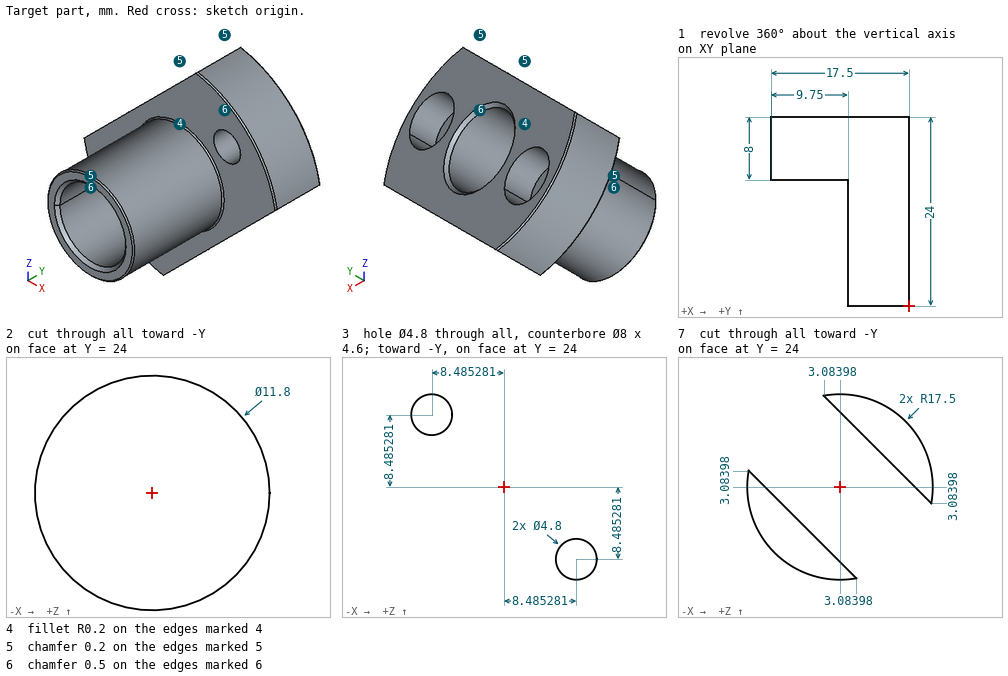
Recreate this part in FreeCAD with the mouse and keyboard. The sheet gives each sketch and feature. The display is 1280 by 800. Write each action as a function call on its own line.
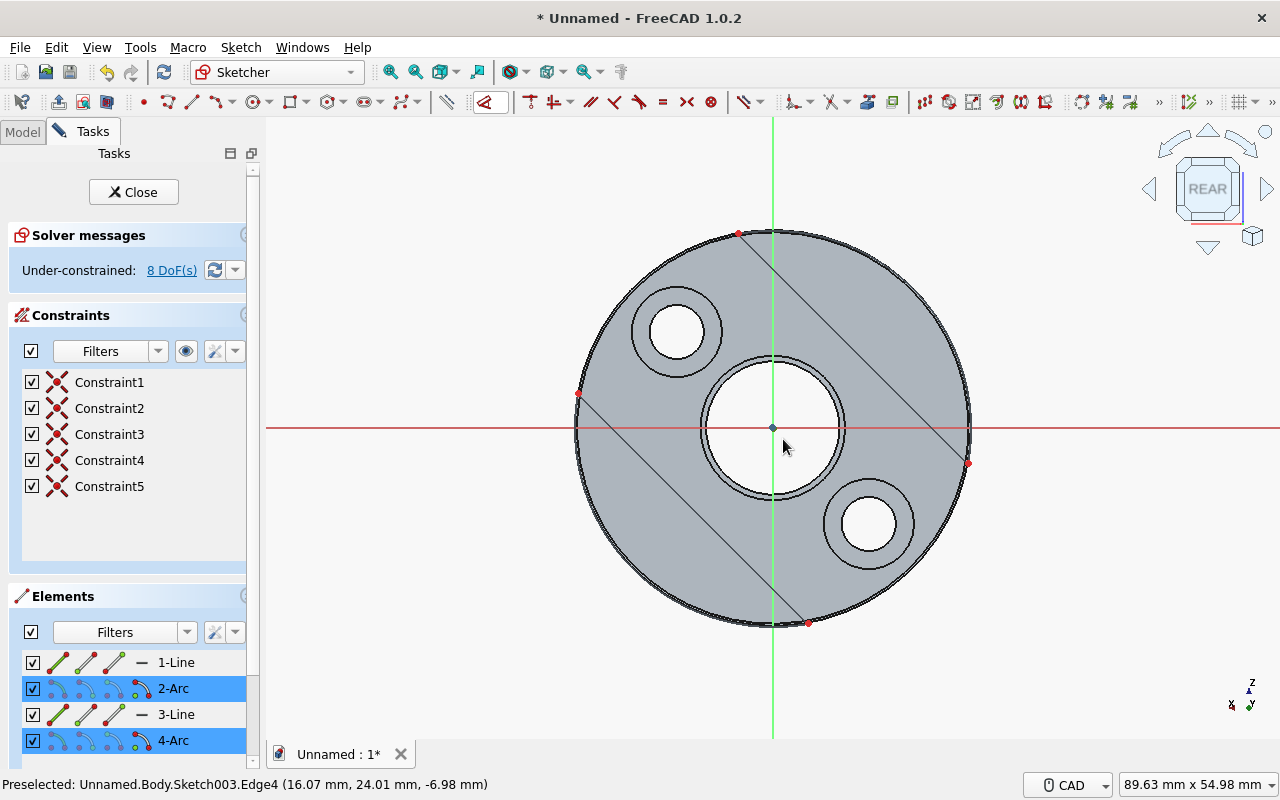
key(c)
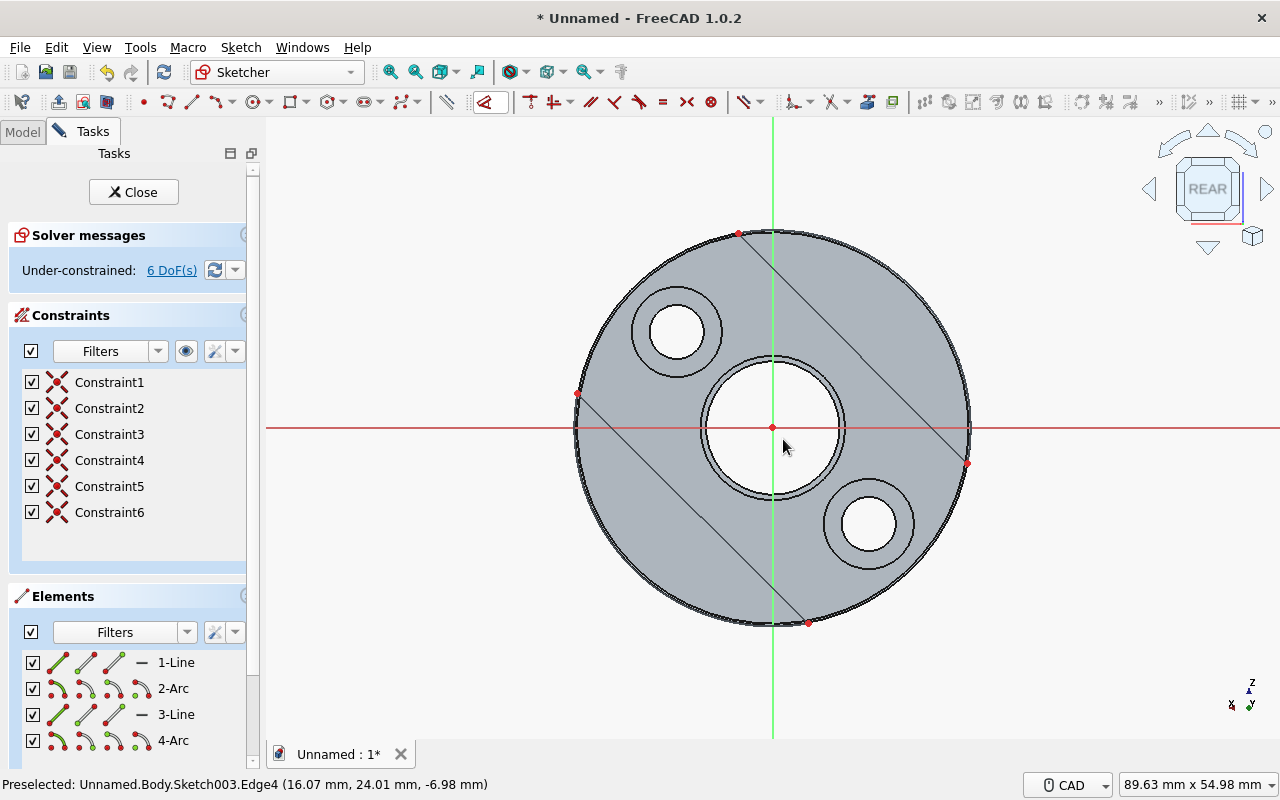
click(955, 352)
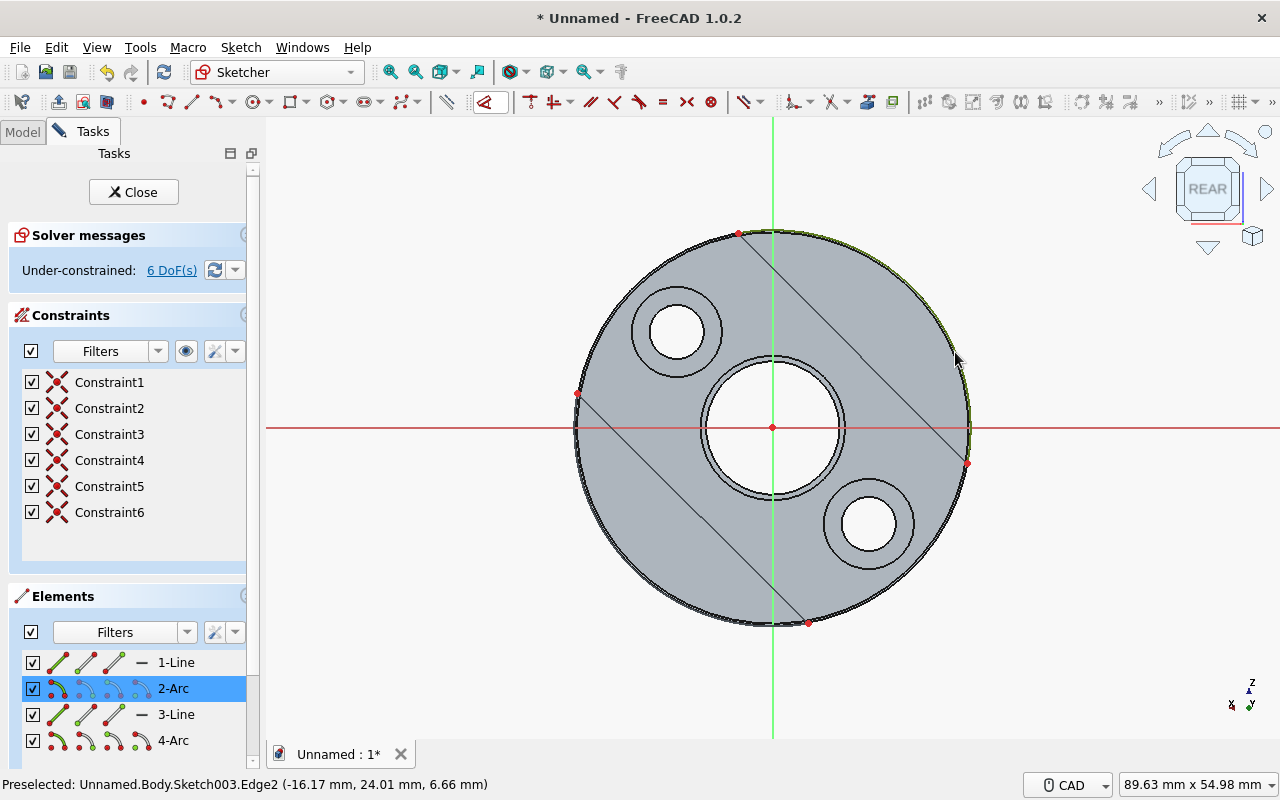
click(590, 506)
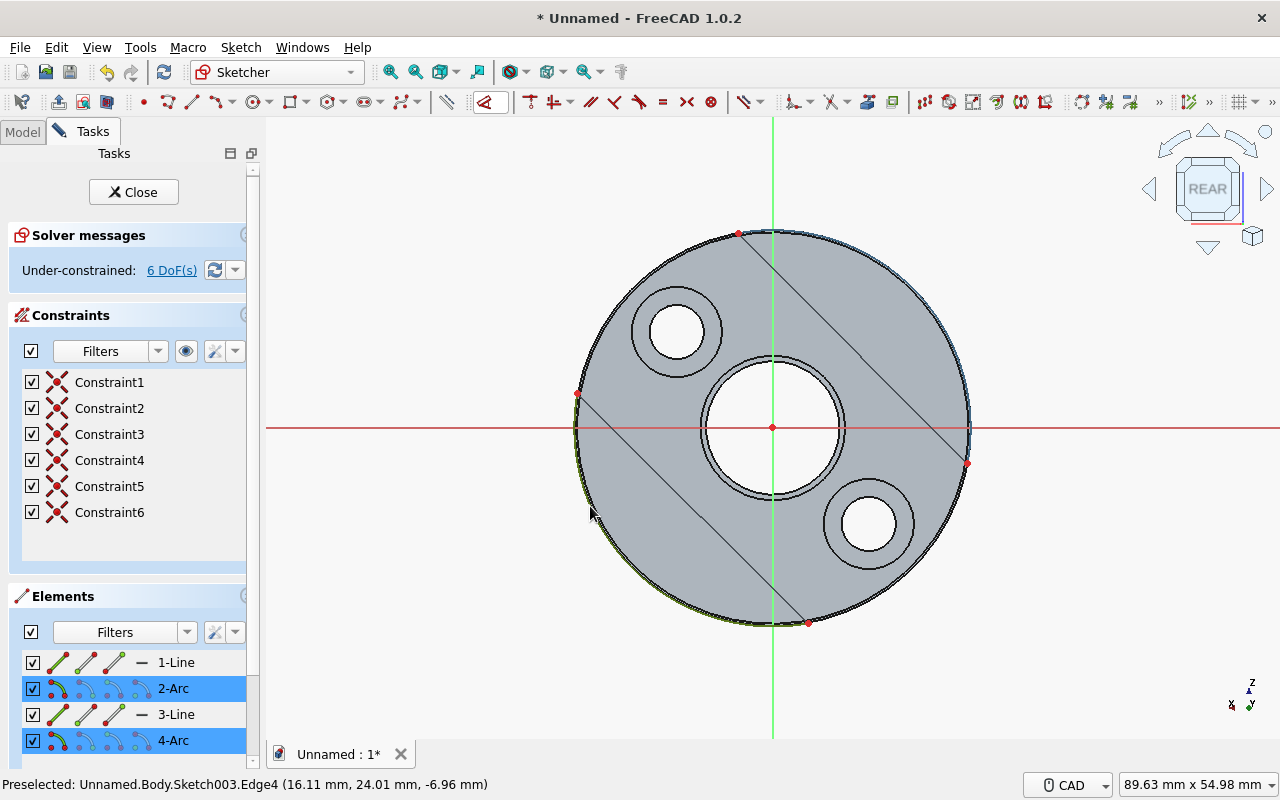
key(e)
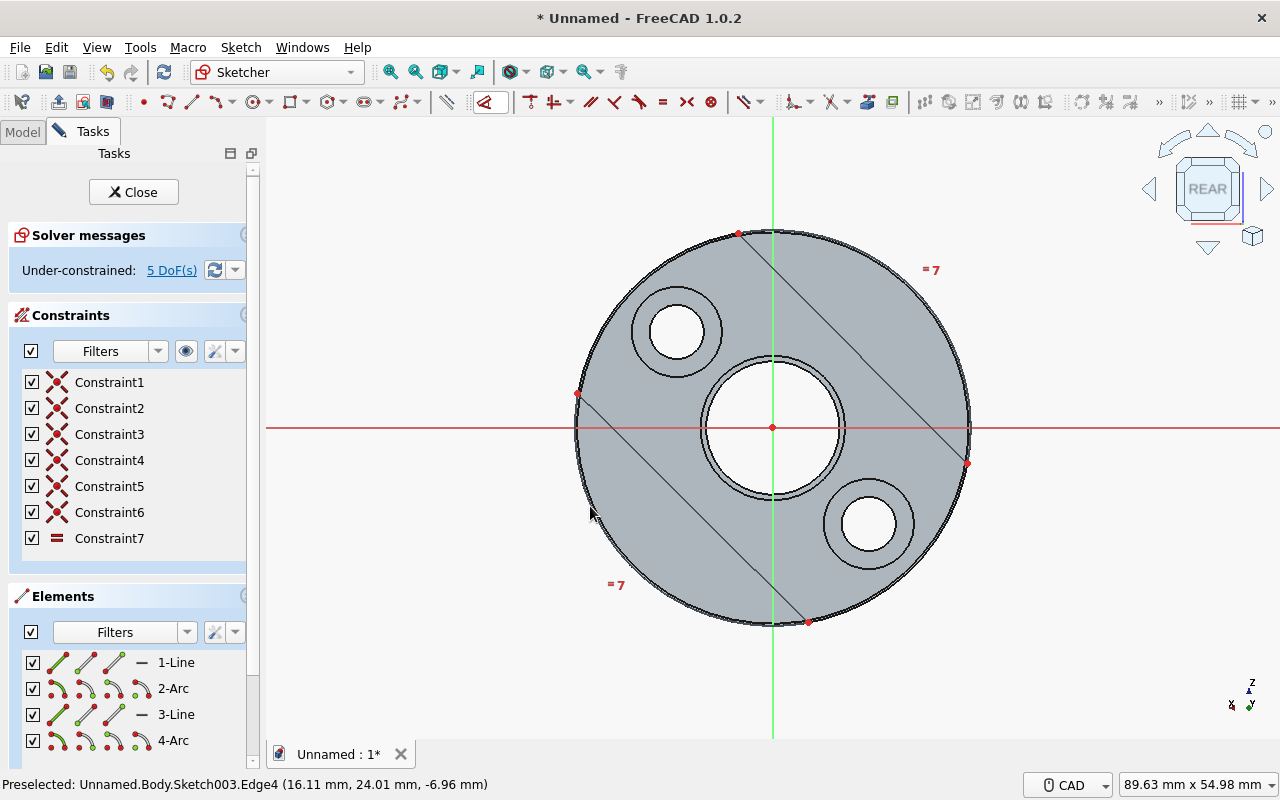
click(955, 352)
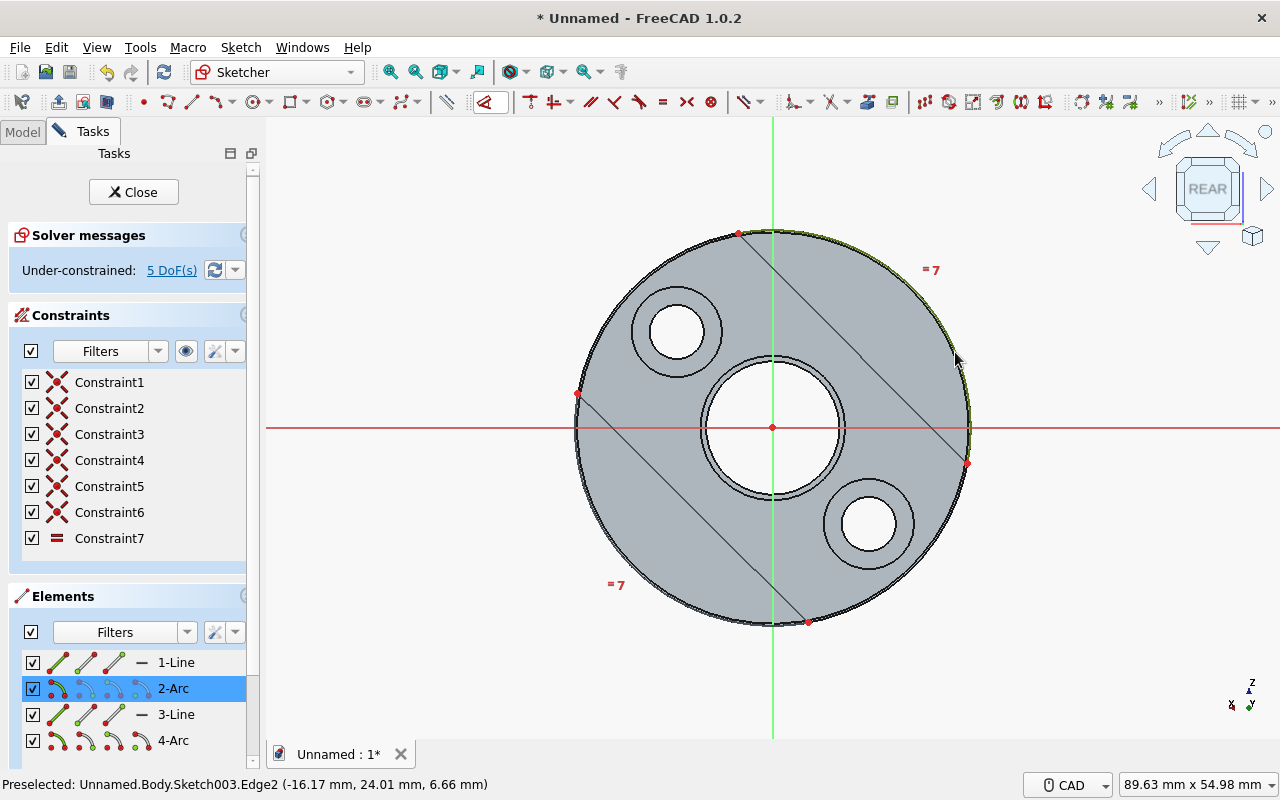
key(k)
key(r)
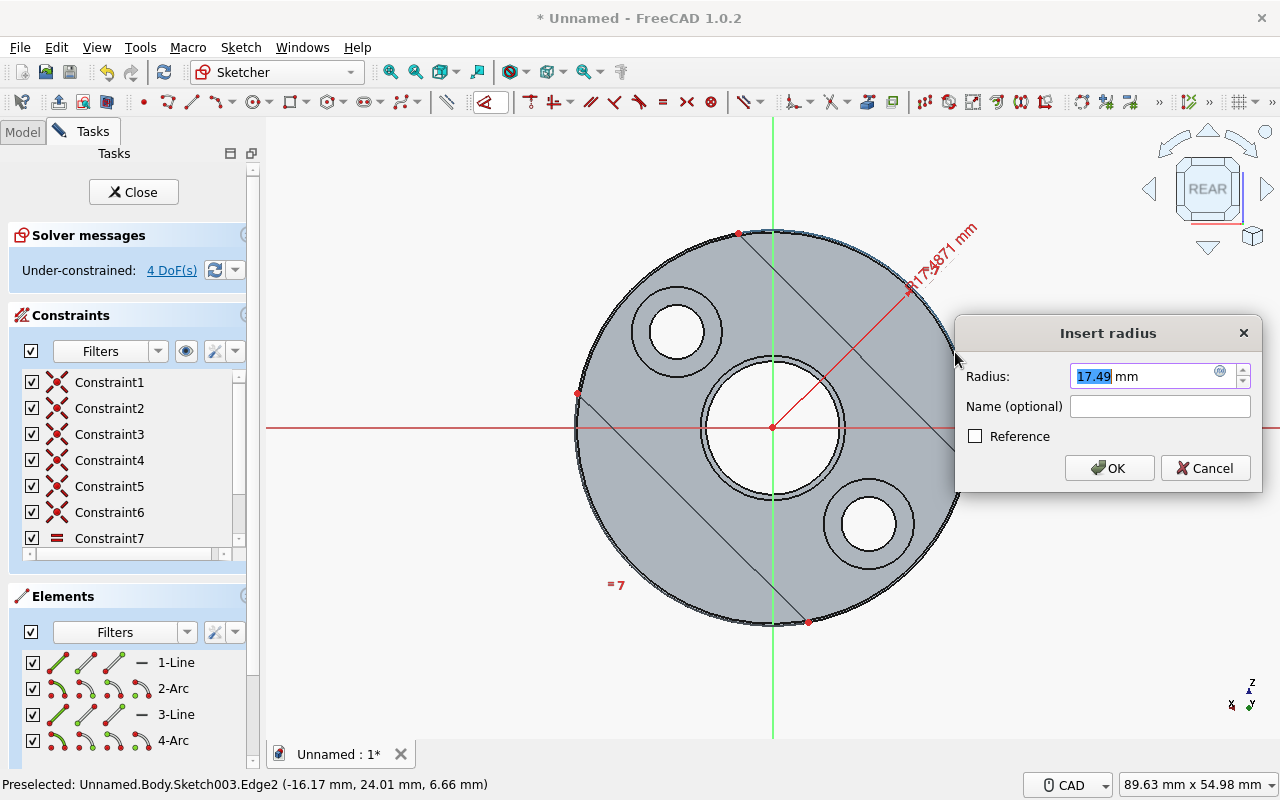
text(17.5)
key(Return)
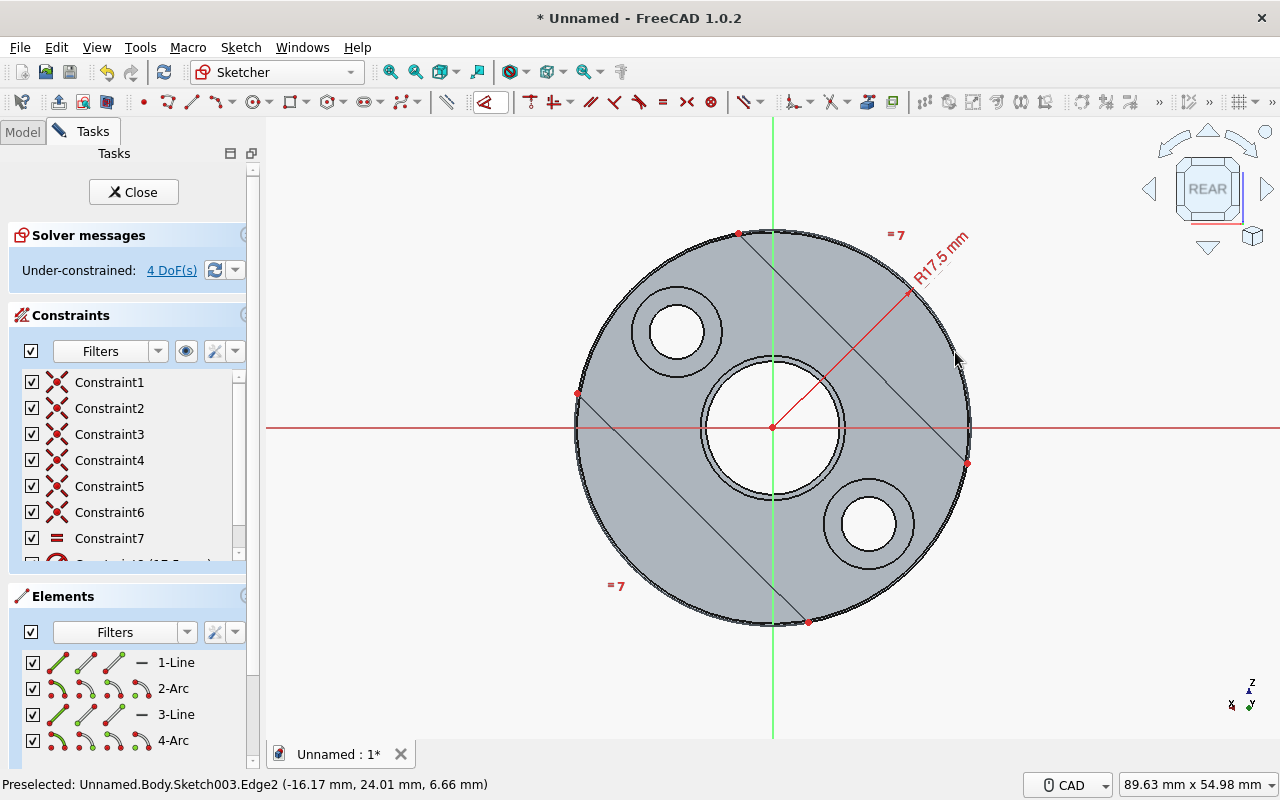
click(738, 233)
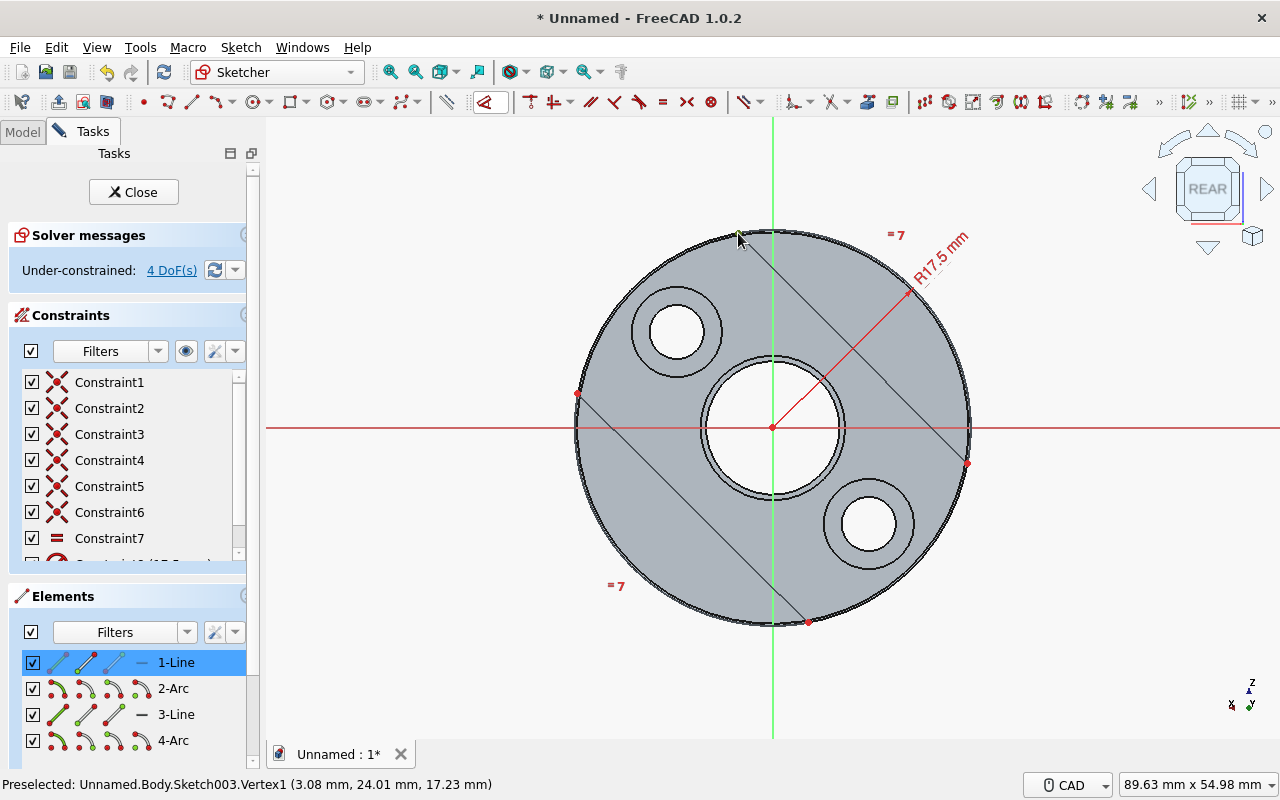
key(l)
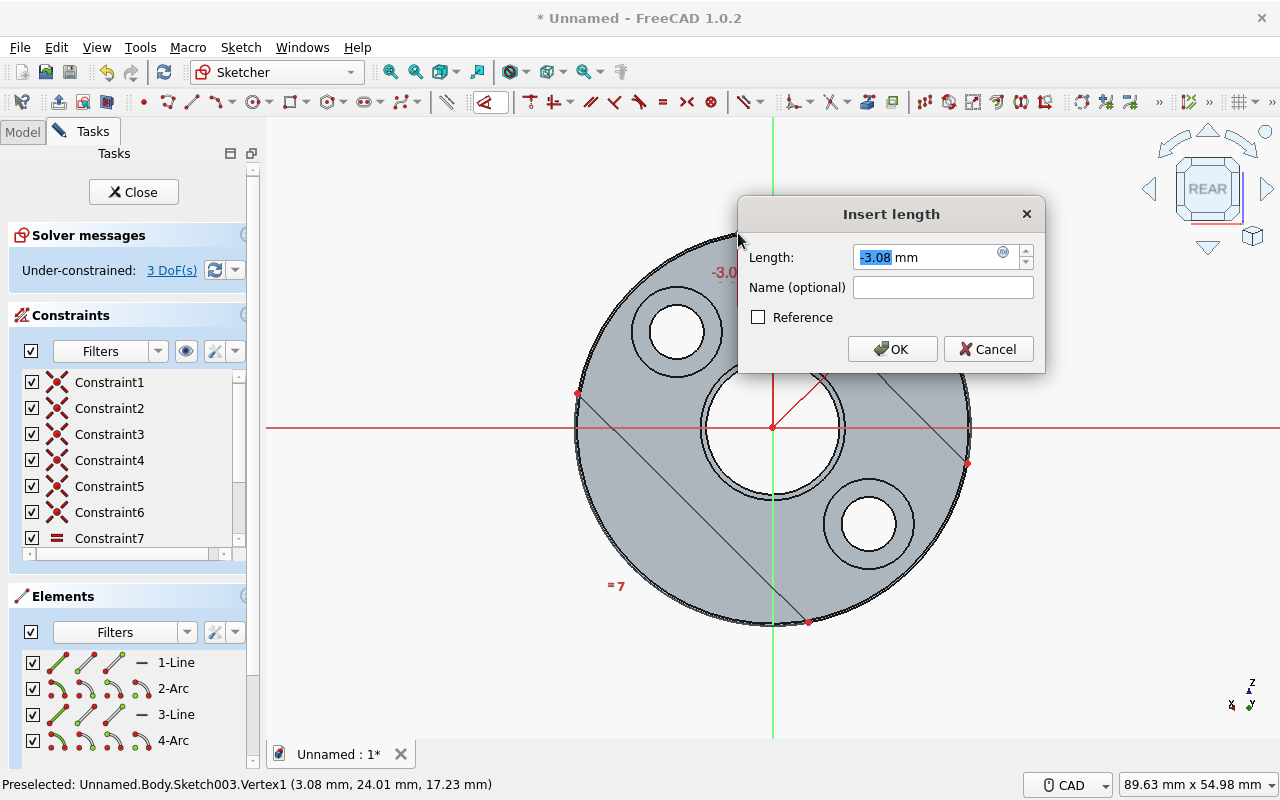
text(-3.08398)
key(Return)